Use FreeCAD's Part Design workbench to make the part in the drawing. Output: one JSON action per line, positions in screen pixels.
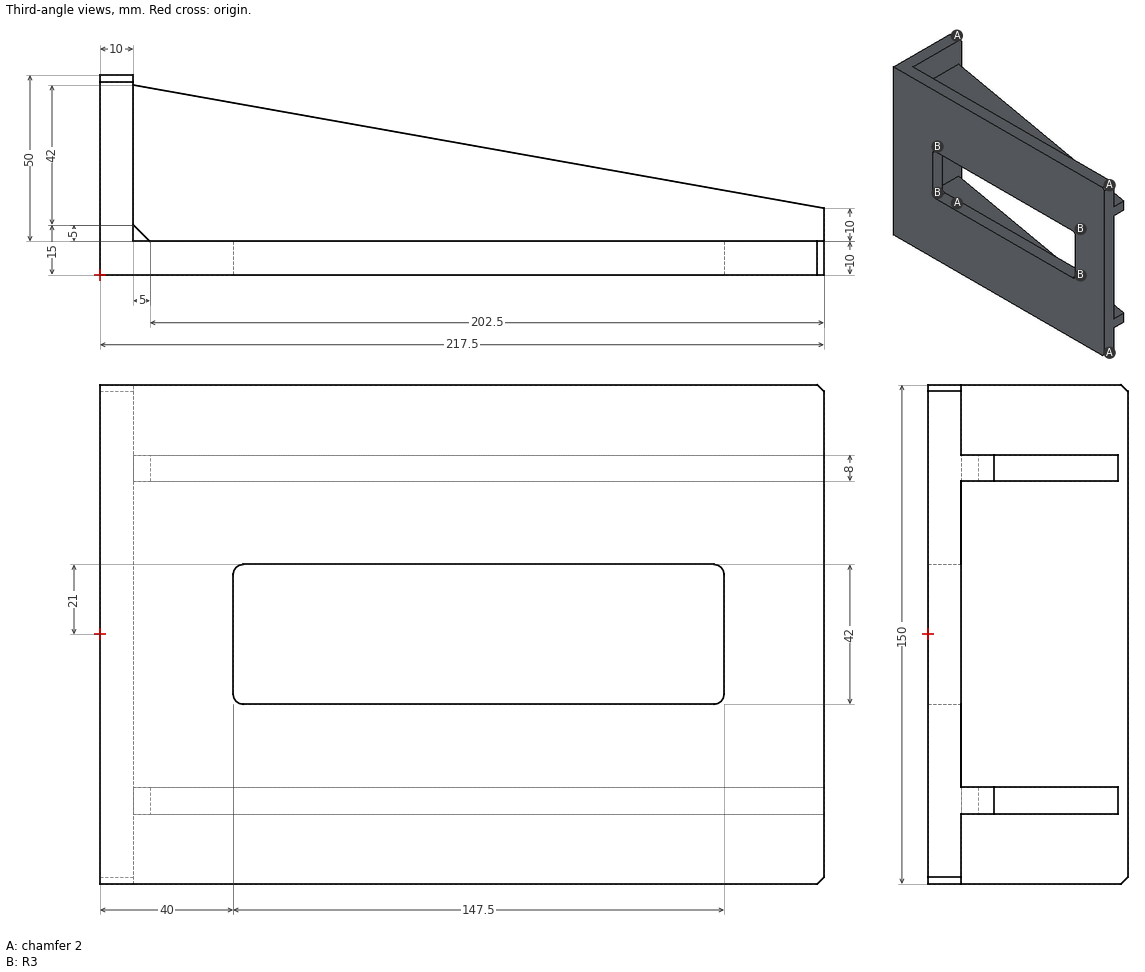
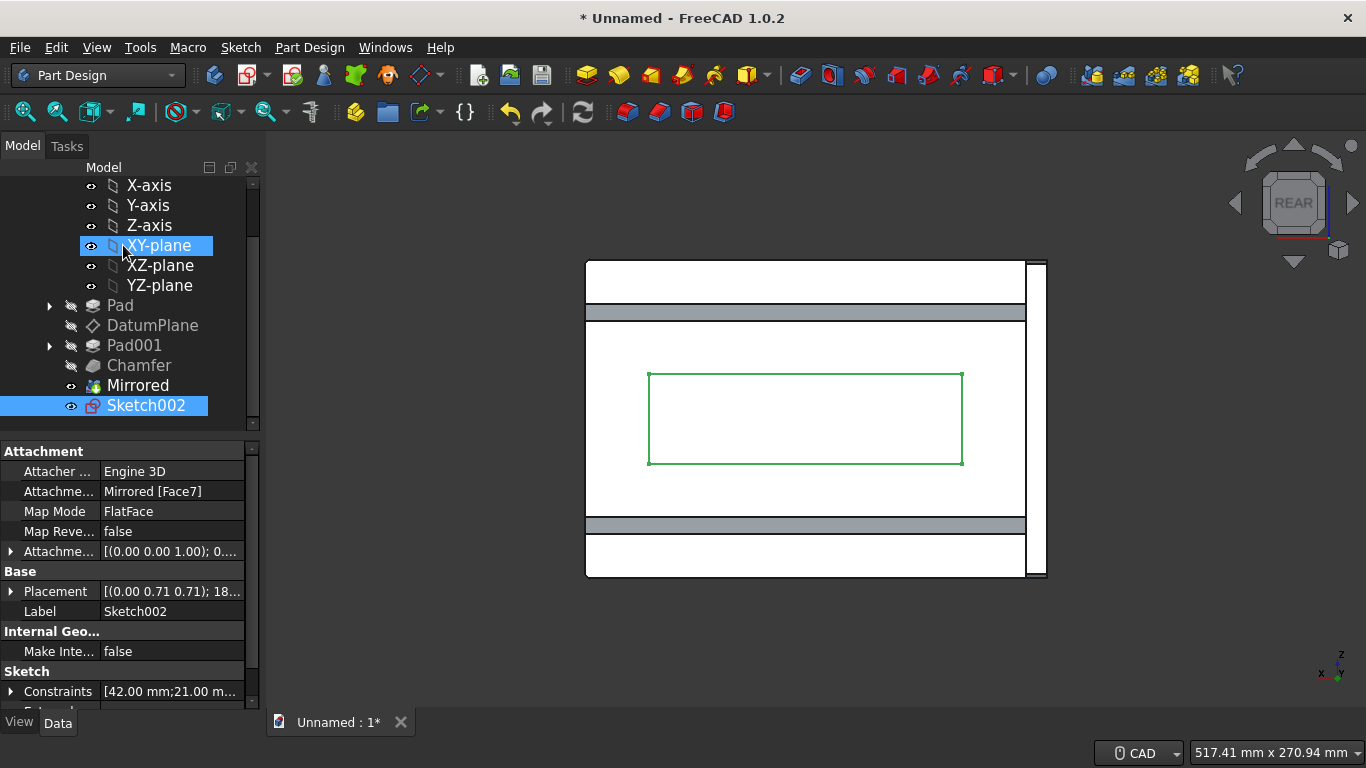
{"action": "left_click", "coordinate": [802, 76]}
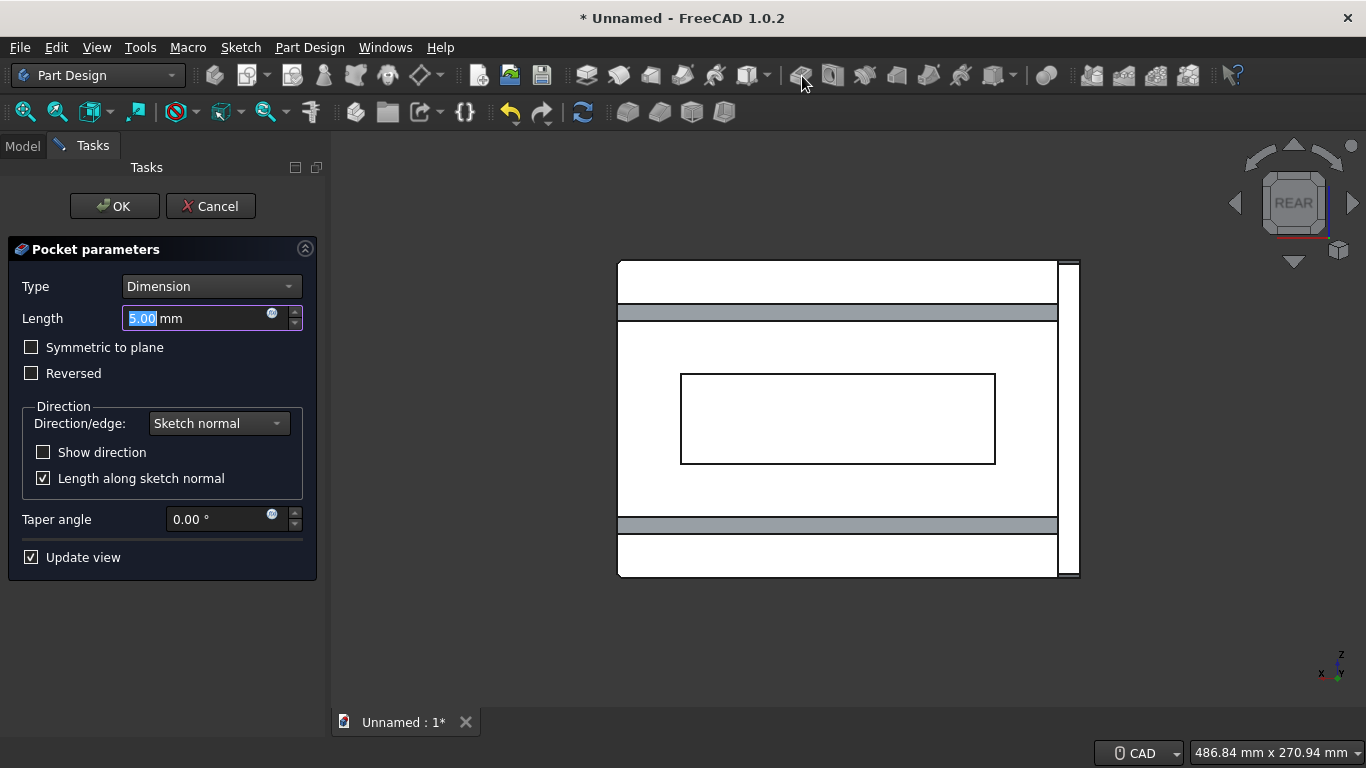
{"action": "left_click", "coordinate": [212, 286]}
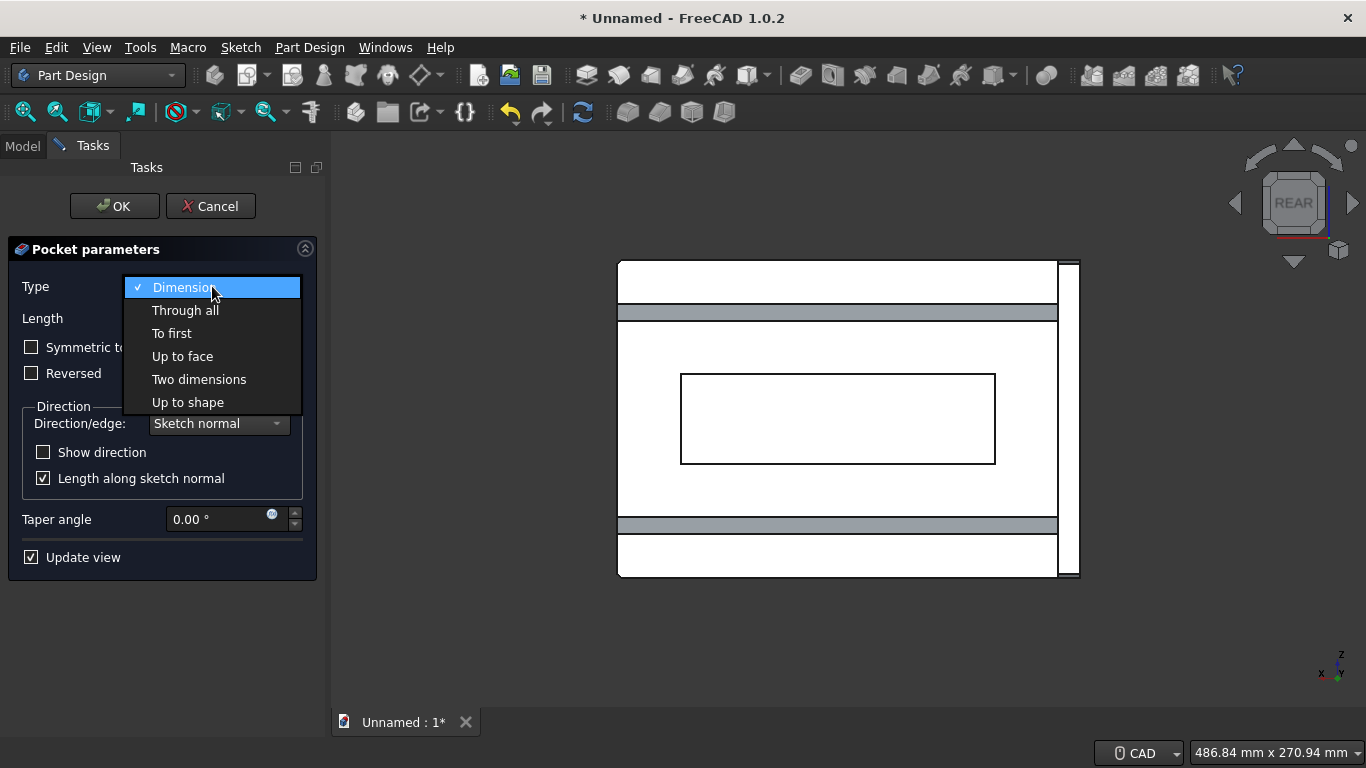
{"action": "left_click", "coordinate": [212, 334]}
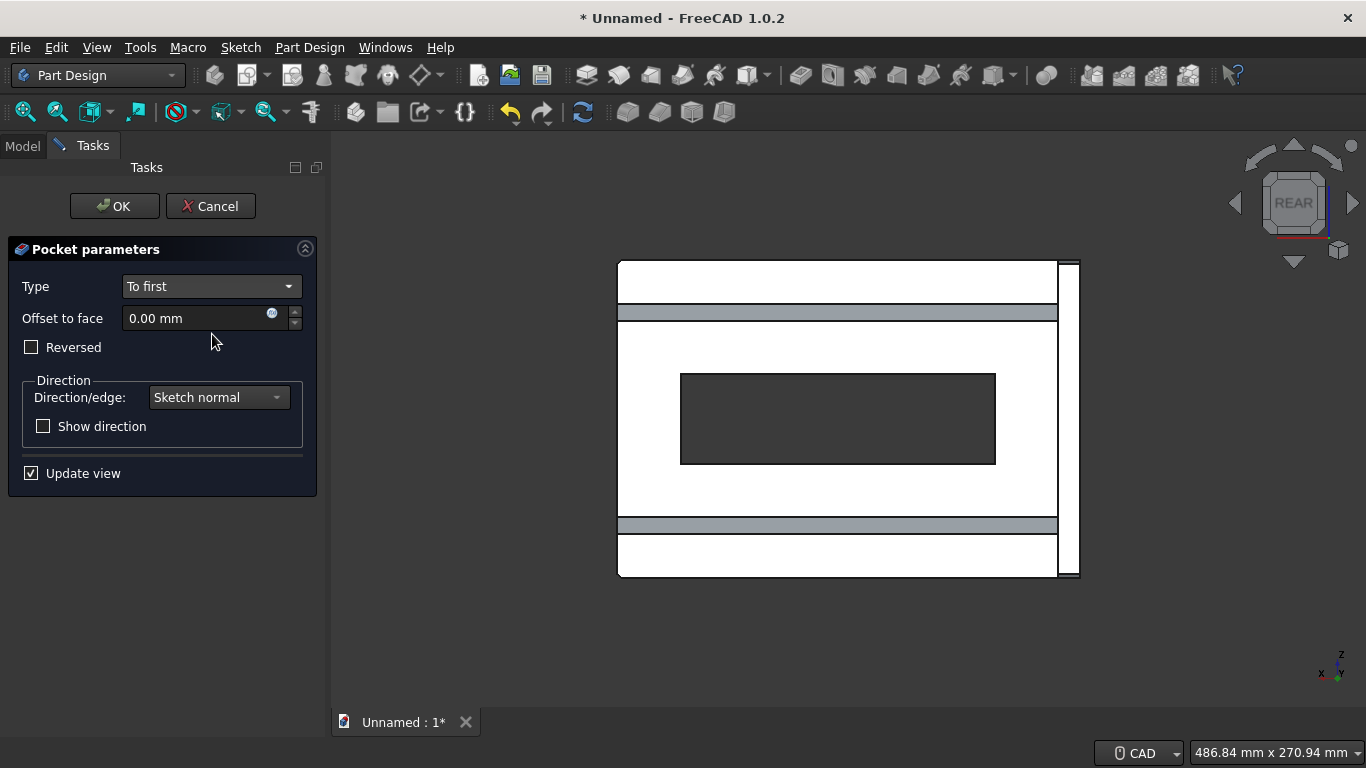
{"action": "left_click", "coordinate": [115, 206]}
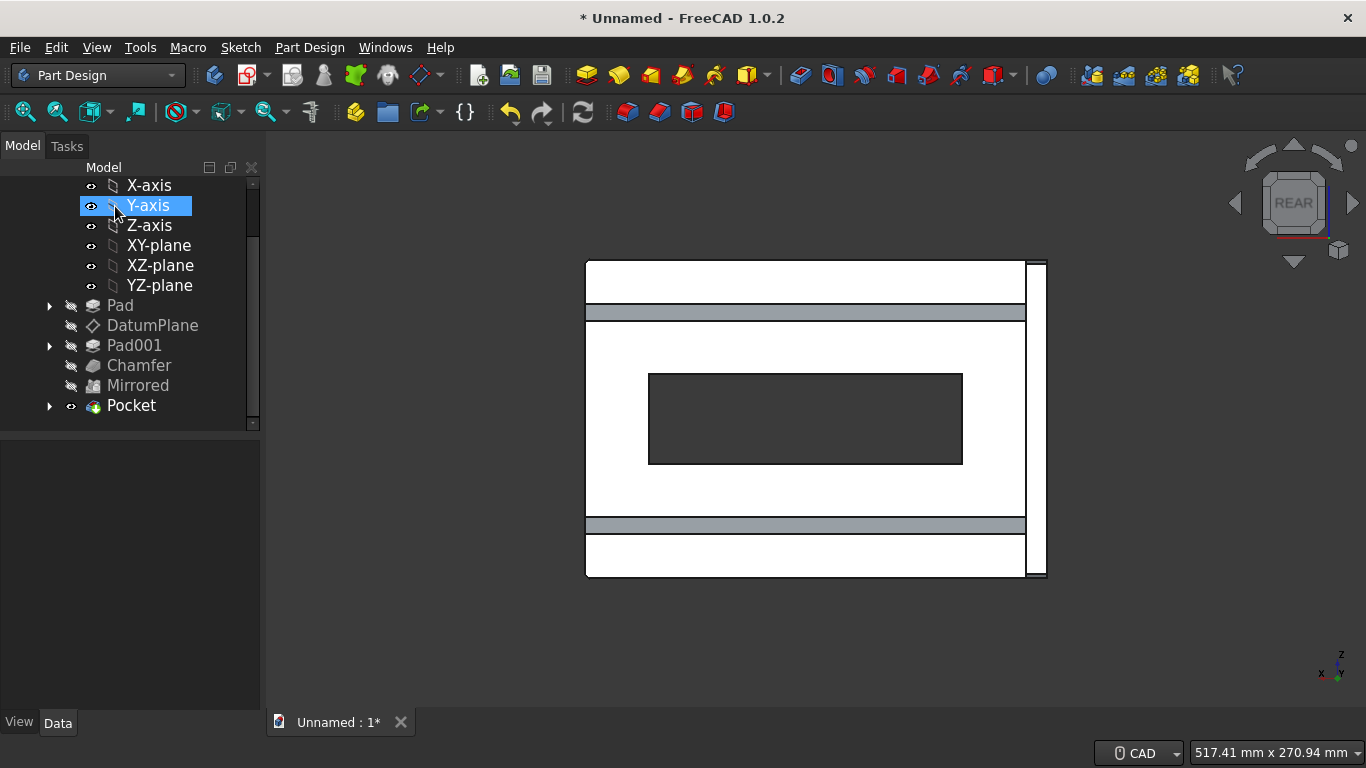
{"action": "scroll", "coordinate": [649, 463], "scroll_direction": "up", "scroll_amount": 4}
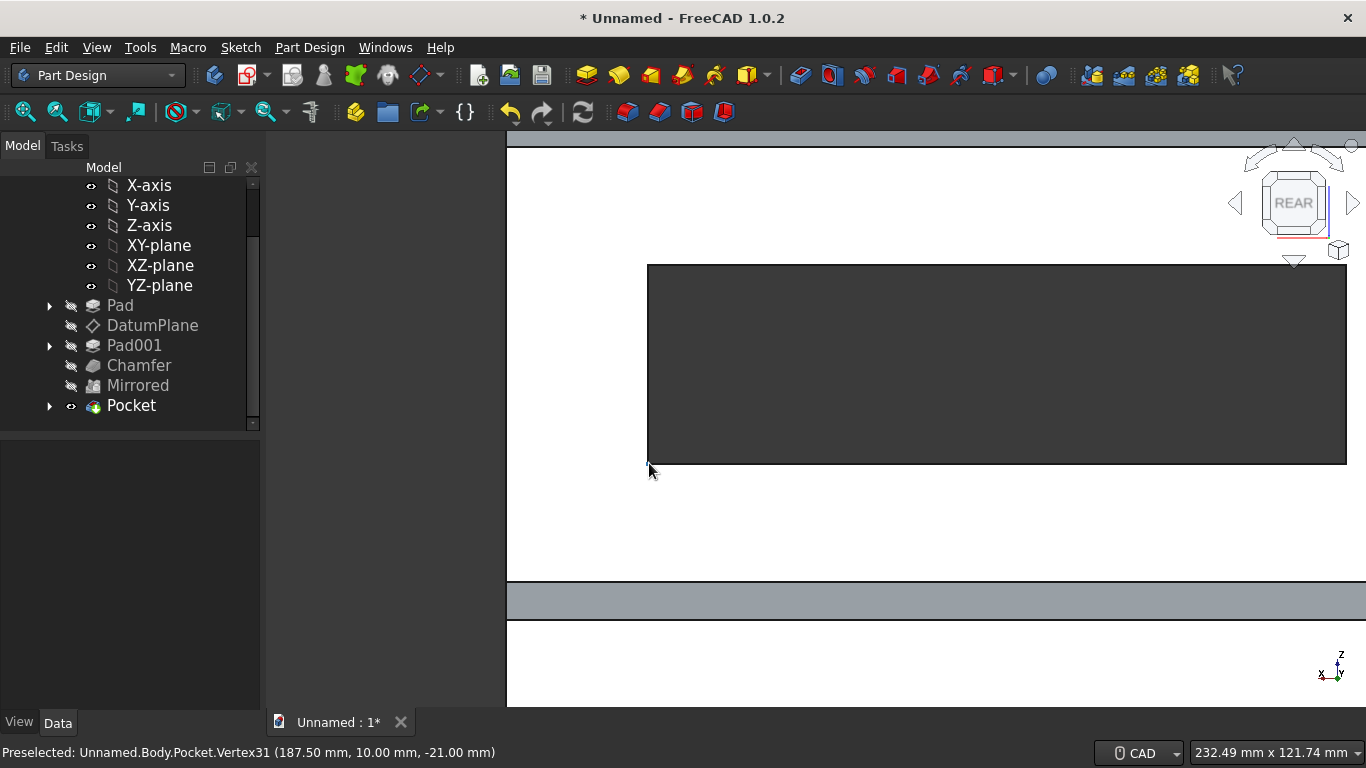
{"action": "left_click", "coordinate": [26, 112]}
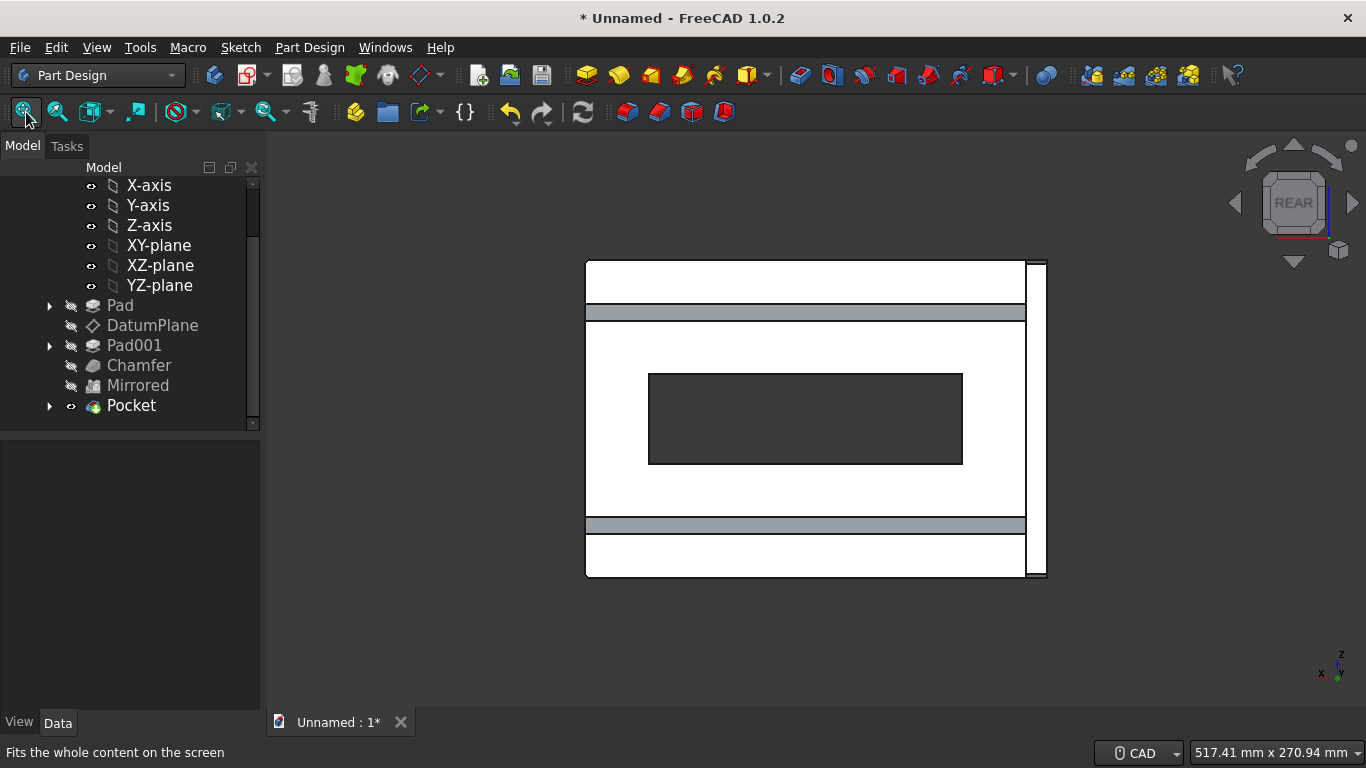
{"action": "key", "text": "0"}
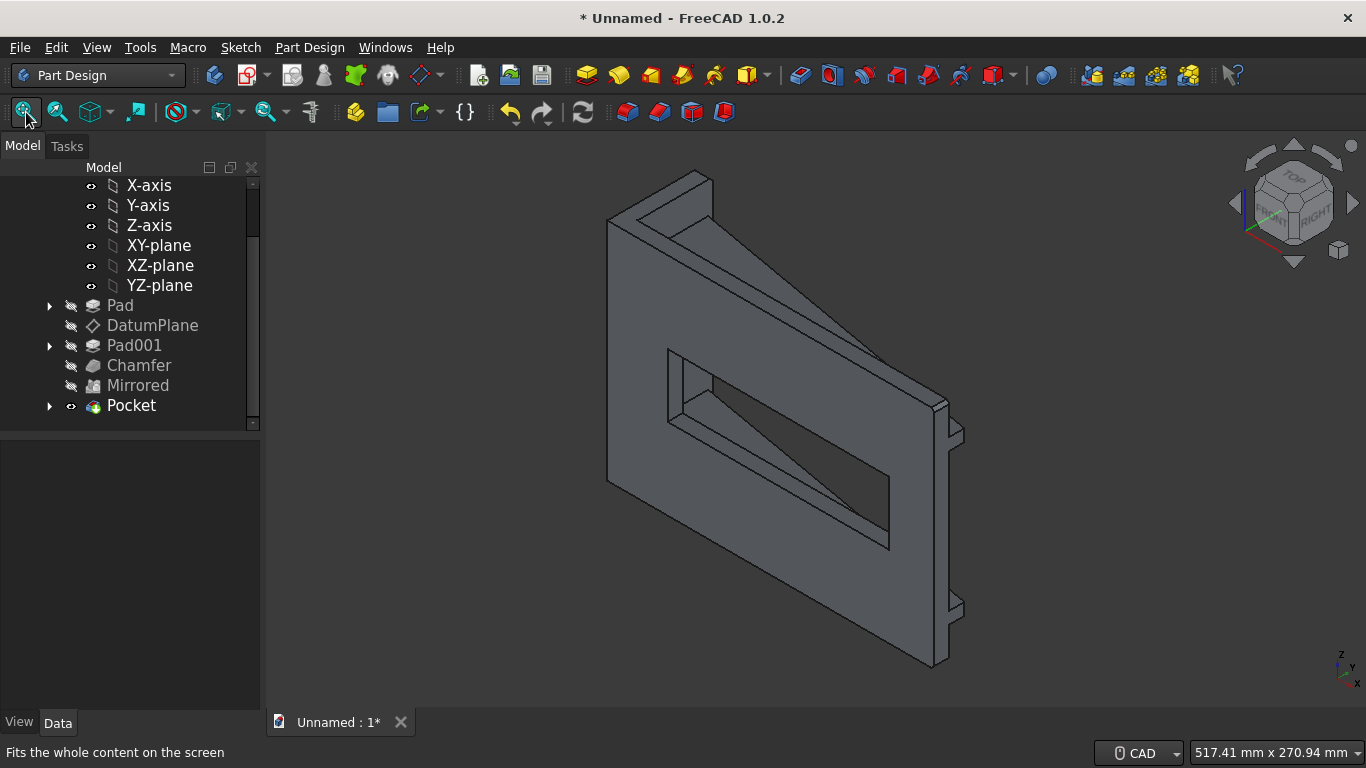
{"action": "scroll", "coordinate": [897, 544], "scroll_direction": "up", "scroll_amount": 4}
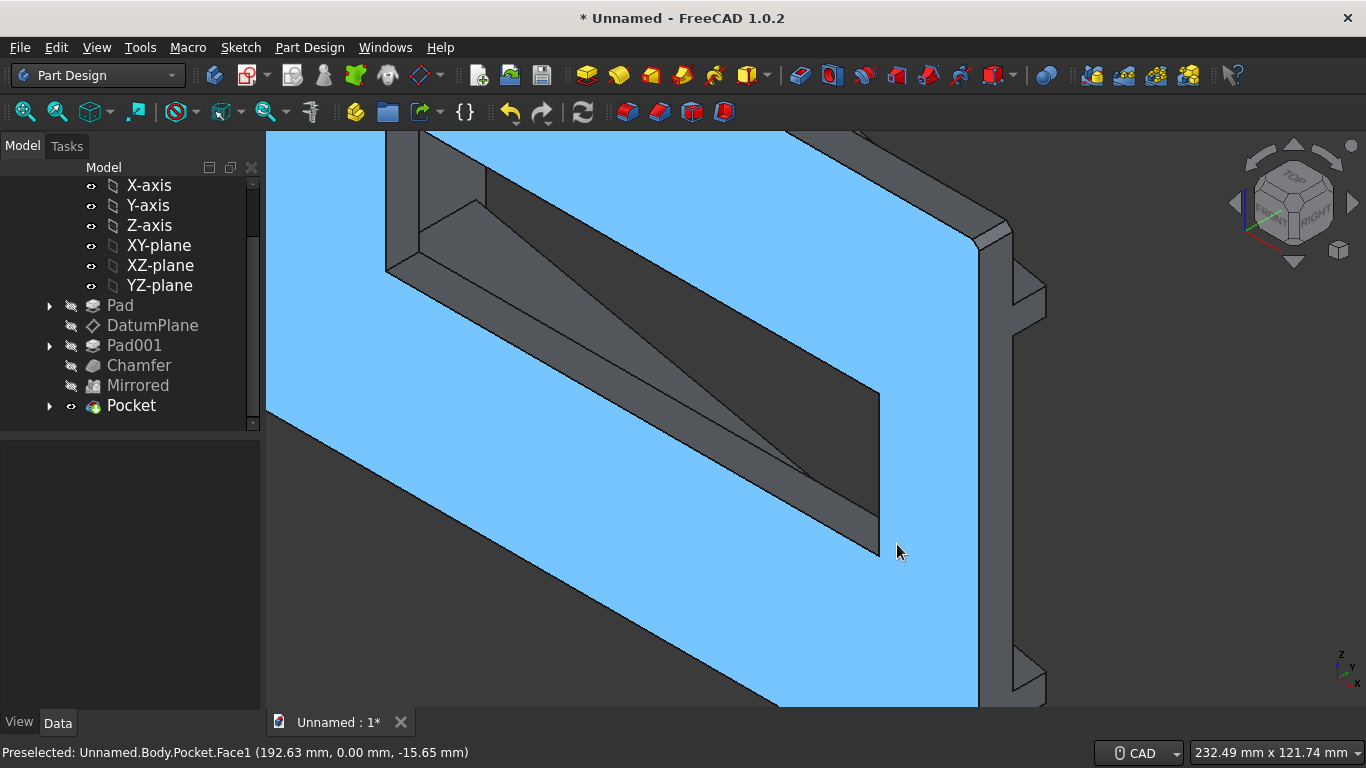
{"action": "left_click", "coordinate": [26, 112]}